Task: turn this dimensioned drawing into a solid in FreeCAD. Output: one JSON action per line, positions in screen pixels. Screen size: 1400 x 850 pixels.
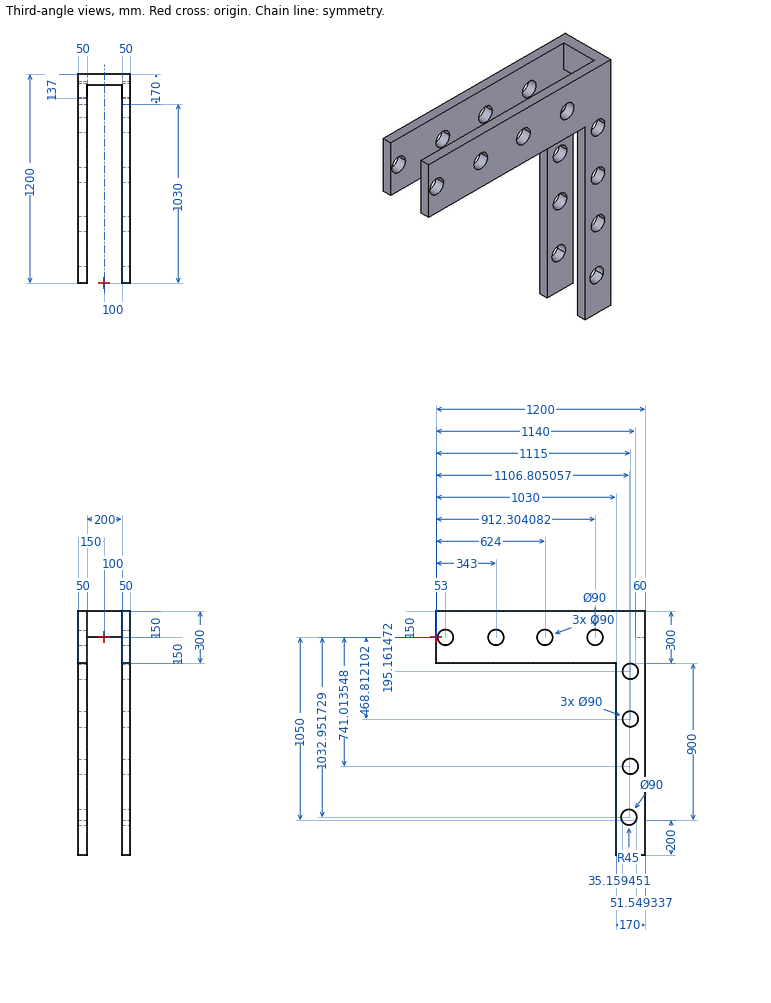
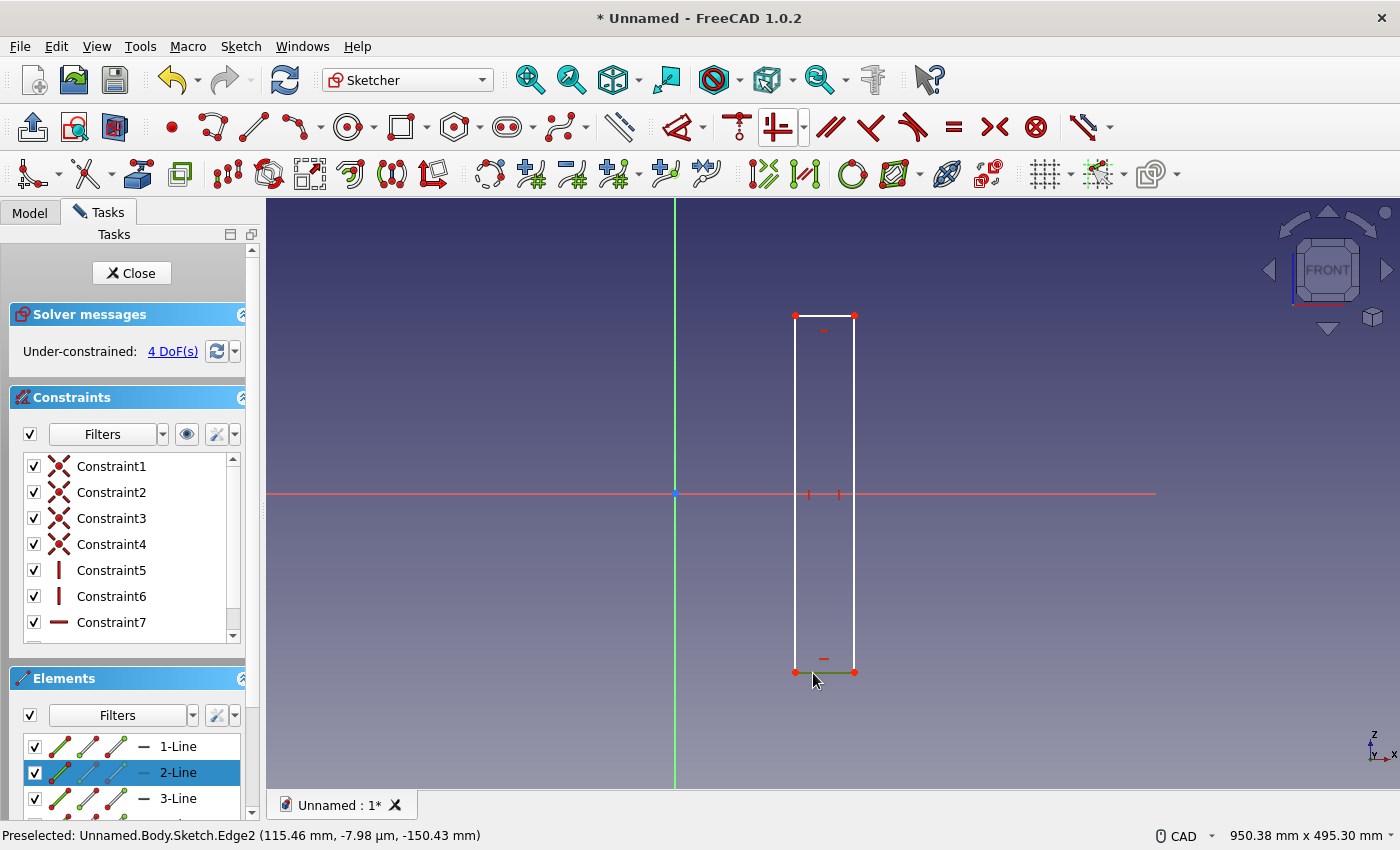
{"action": "left_click", "coordinate": [702, 128]}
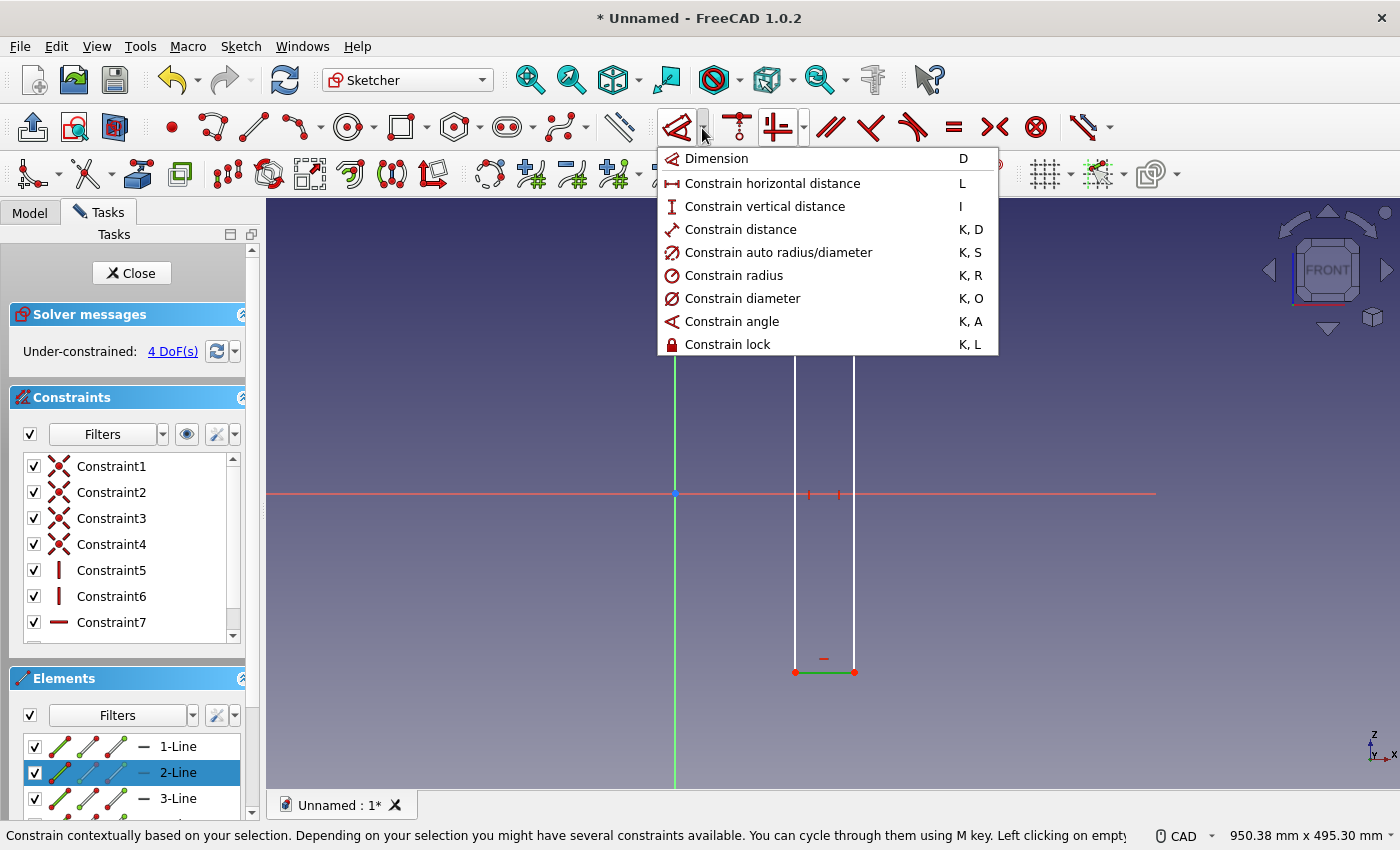
{"action": "left_click", "coordinate": [828, 184]}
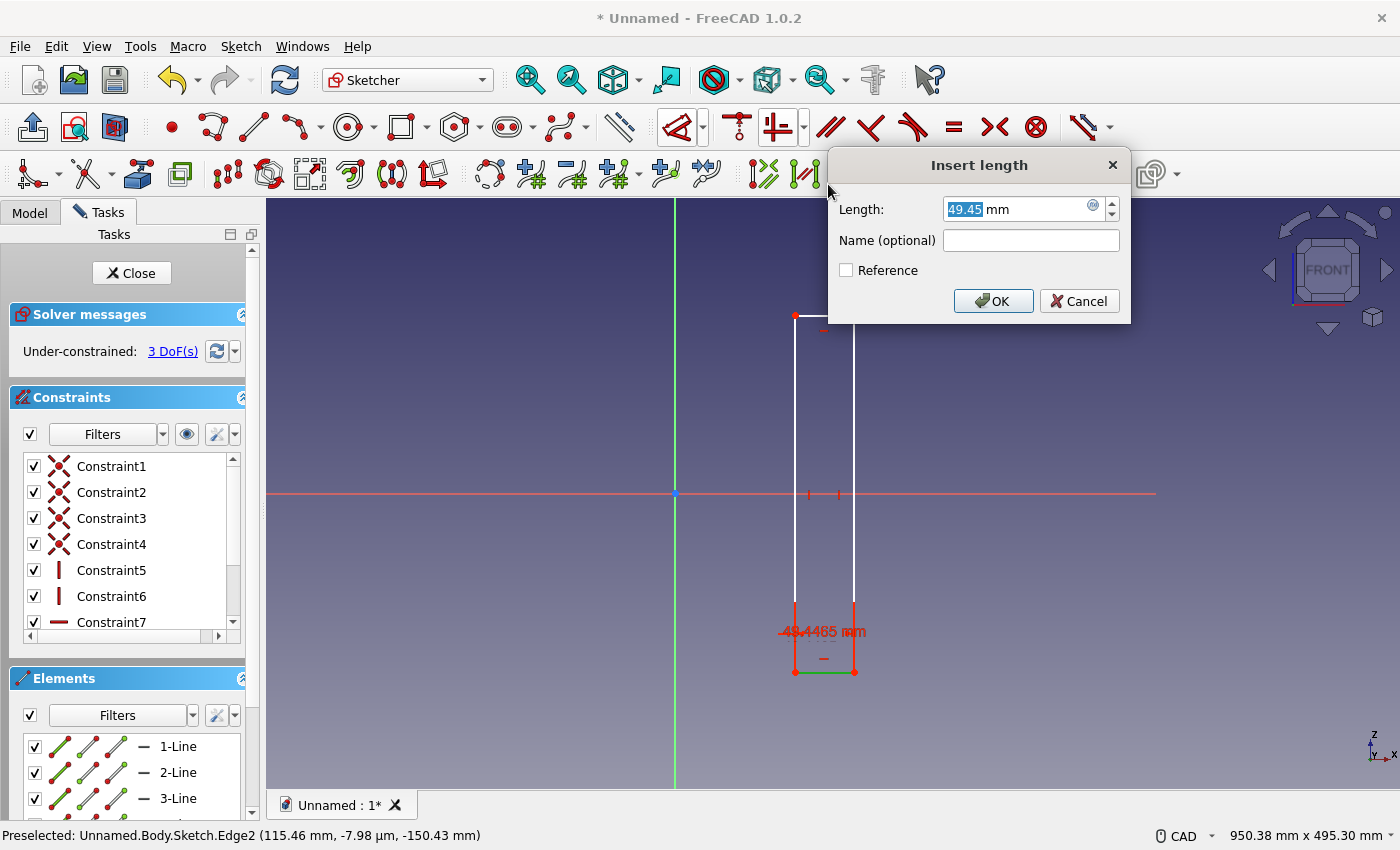
{"action": "type", "text": "50"}
{"action": "key", "text": "Return"}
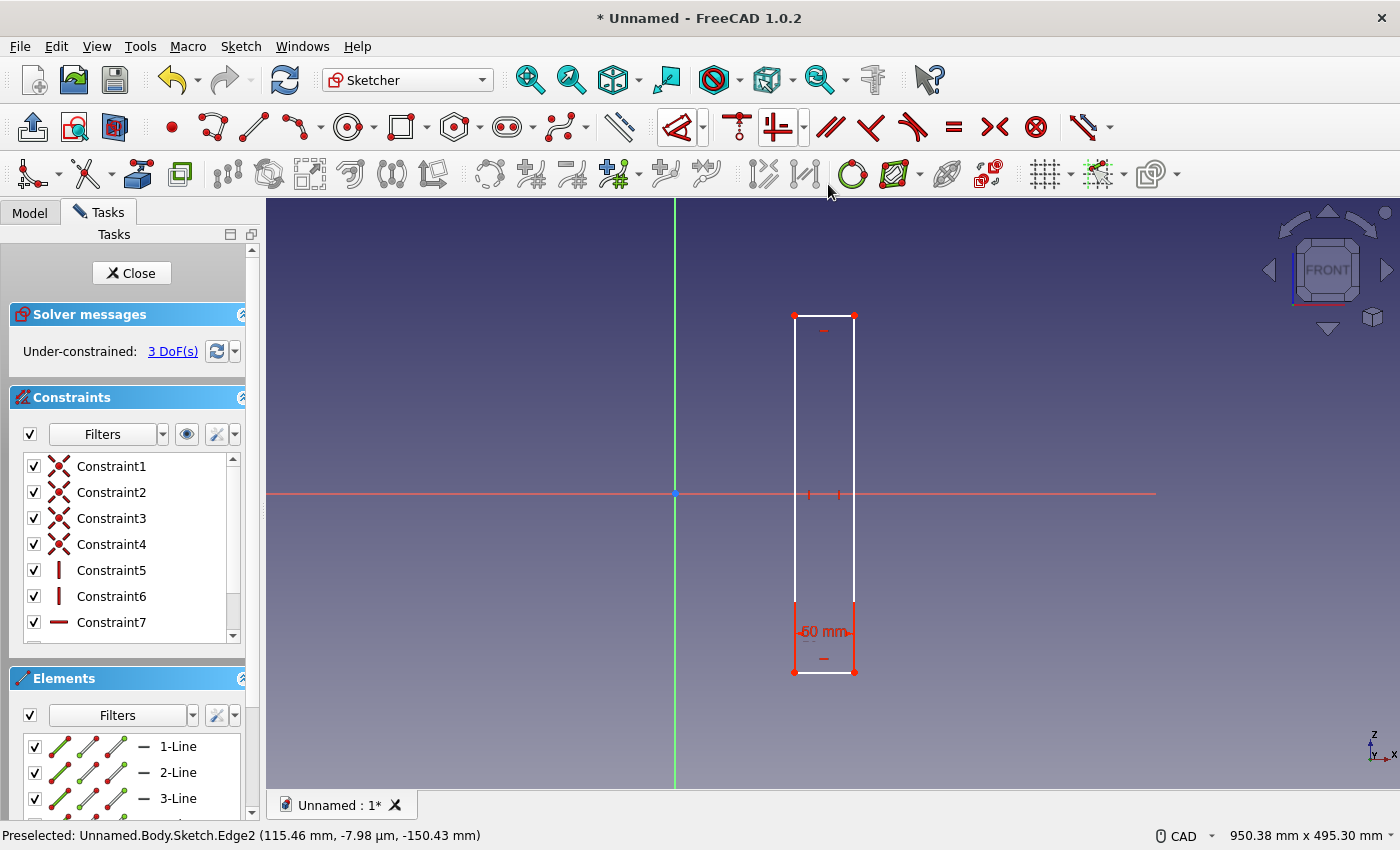
{"action": "left_click", "coordinate": [795, 423]}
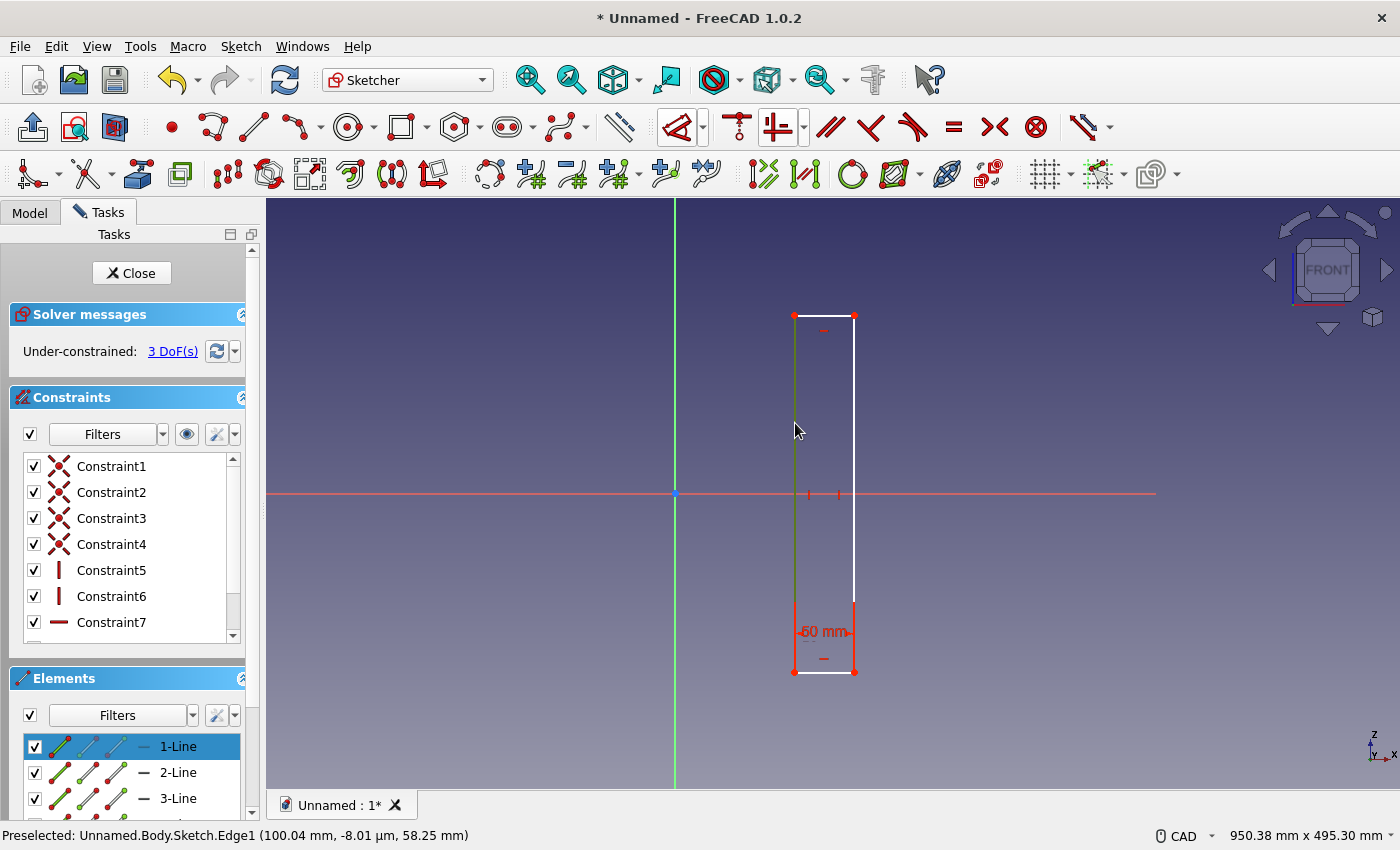
{"action": "key", "text": "i"}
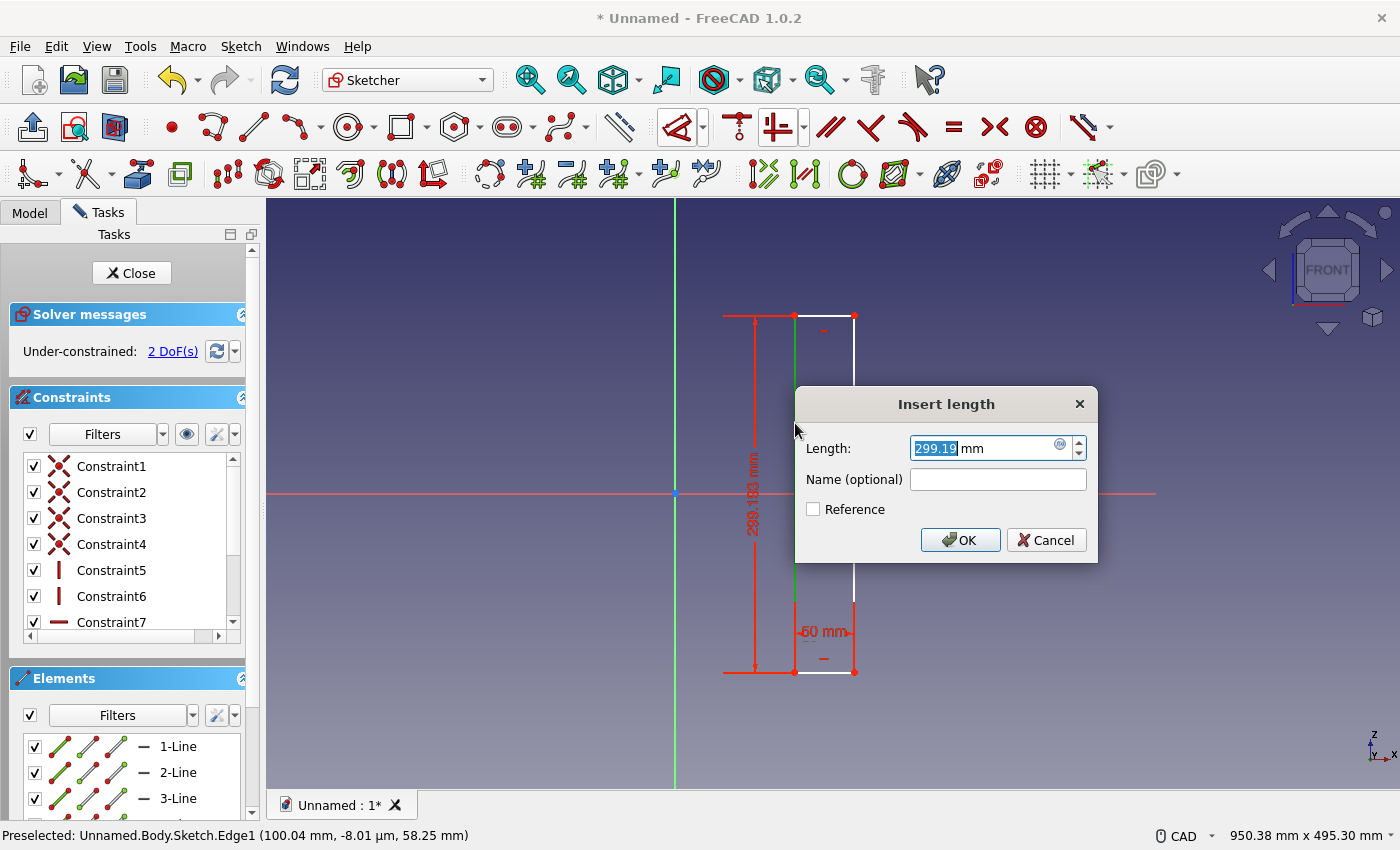
{"action": "type", "text": "300"}
{"action": "key", "text": "Return"}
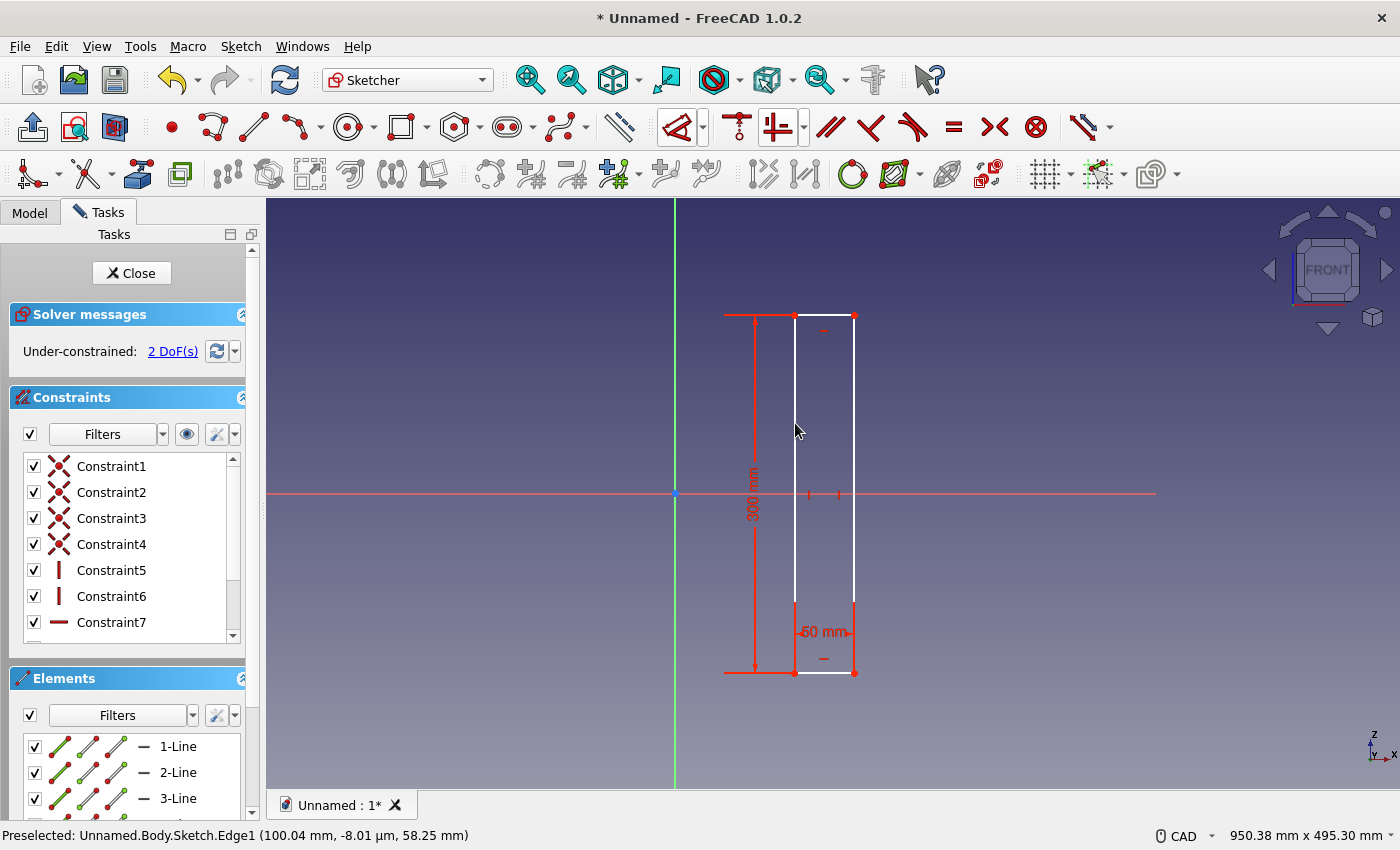
{"action": "left_click", "coordinate": [795, 315]}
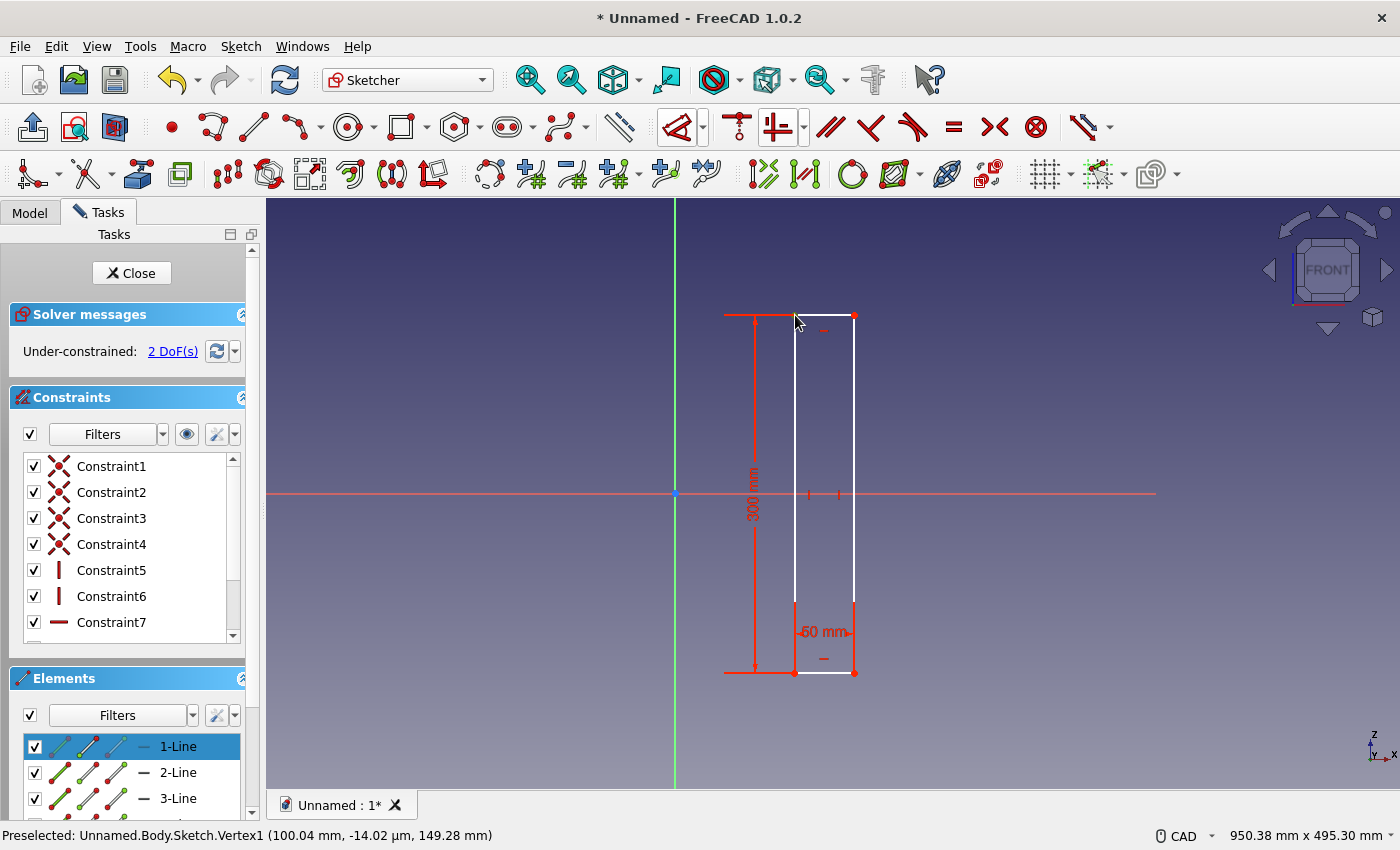
{"action": "left_click", "coordinate": [702, 128]}